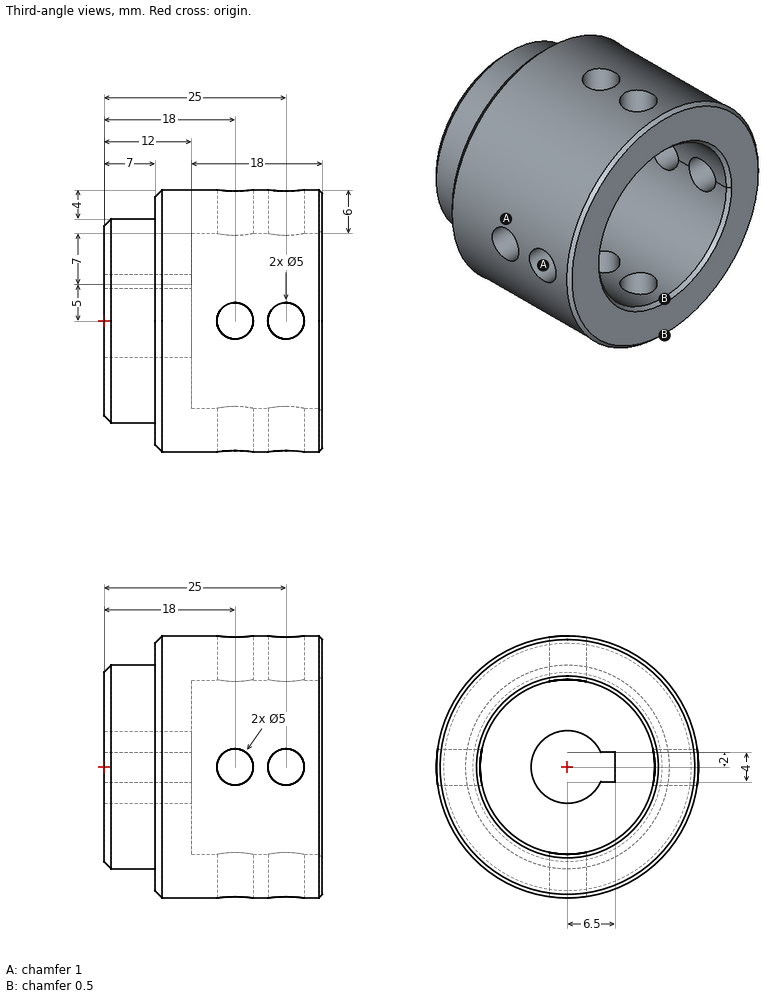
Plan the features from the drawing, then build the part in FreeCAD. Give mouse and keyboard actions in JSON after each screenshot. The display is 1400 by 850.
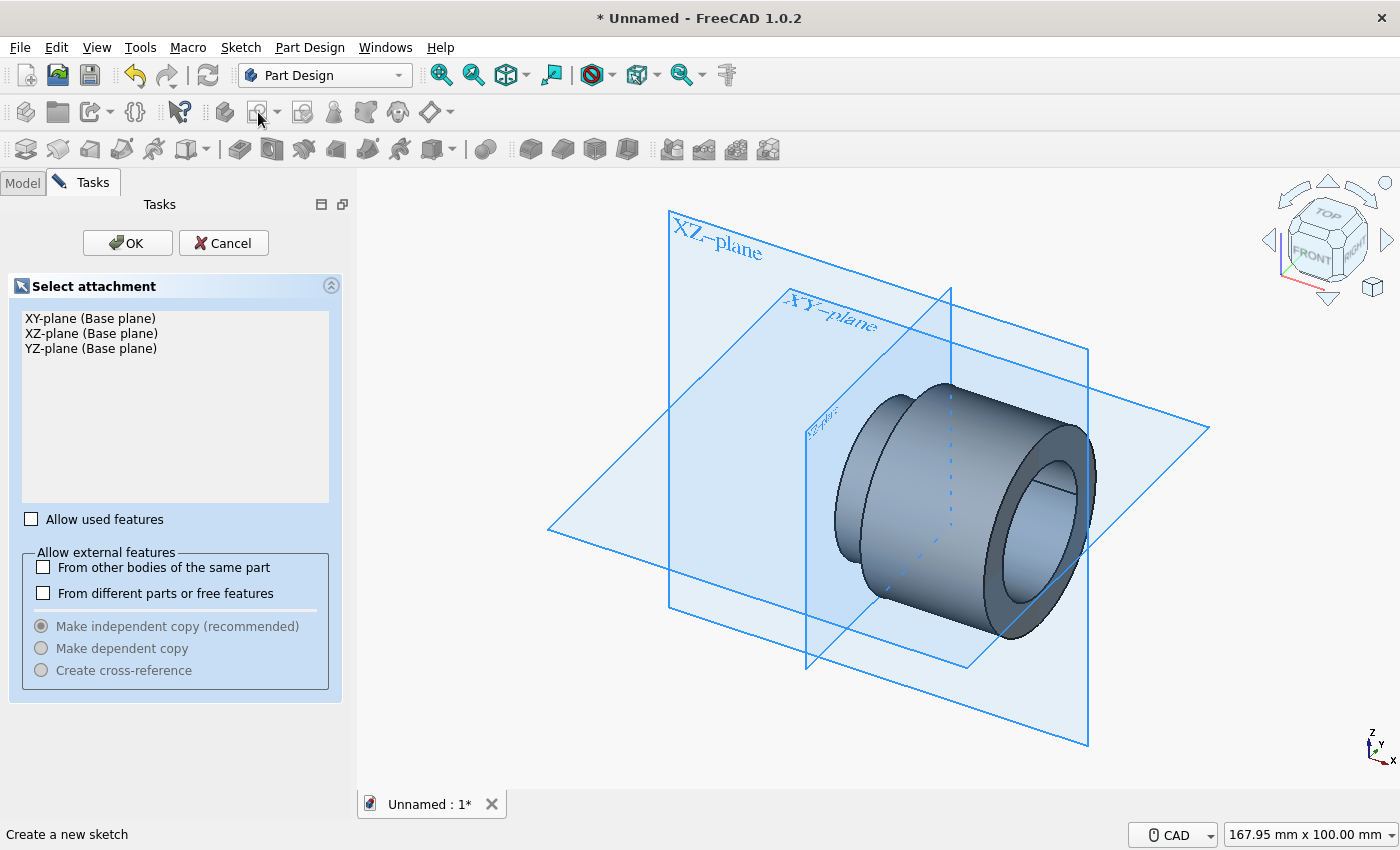
{"action": "left_click", "coordinate": [82, 348]}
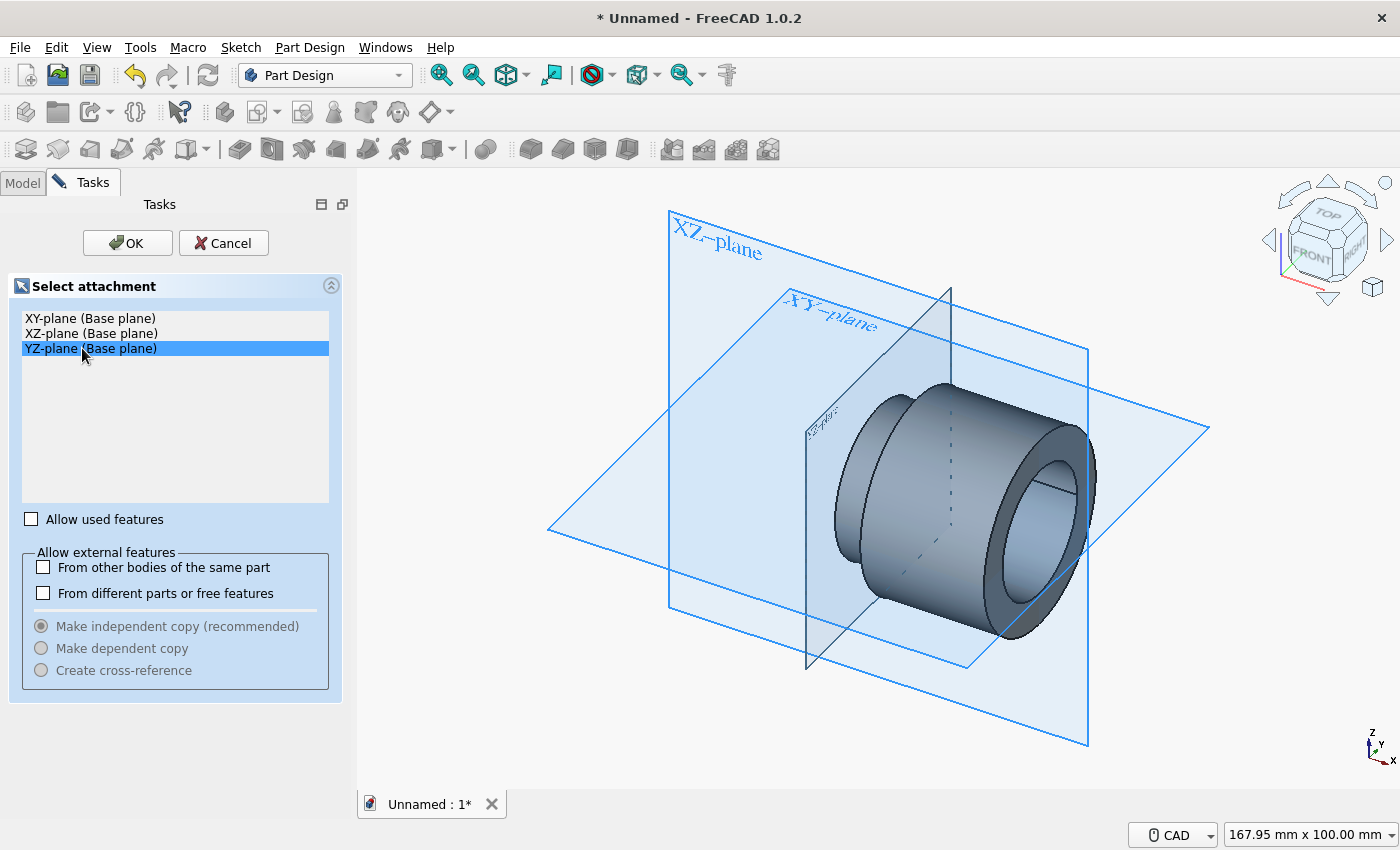
{"action": "left_click", "coordinate": [128, 243]}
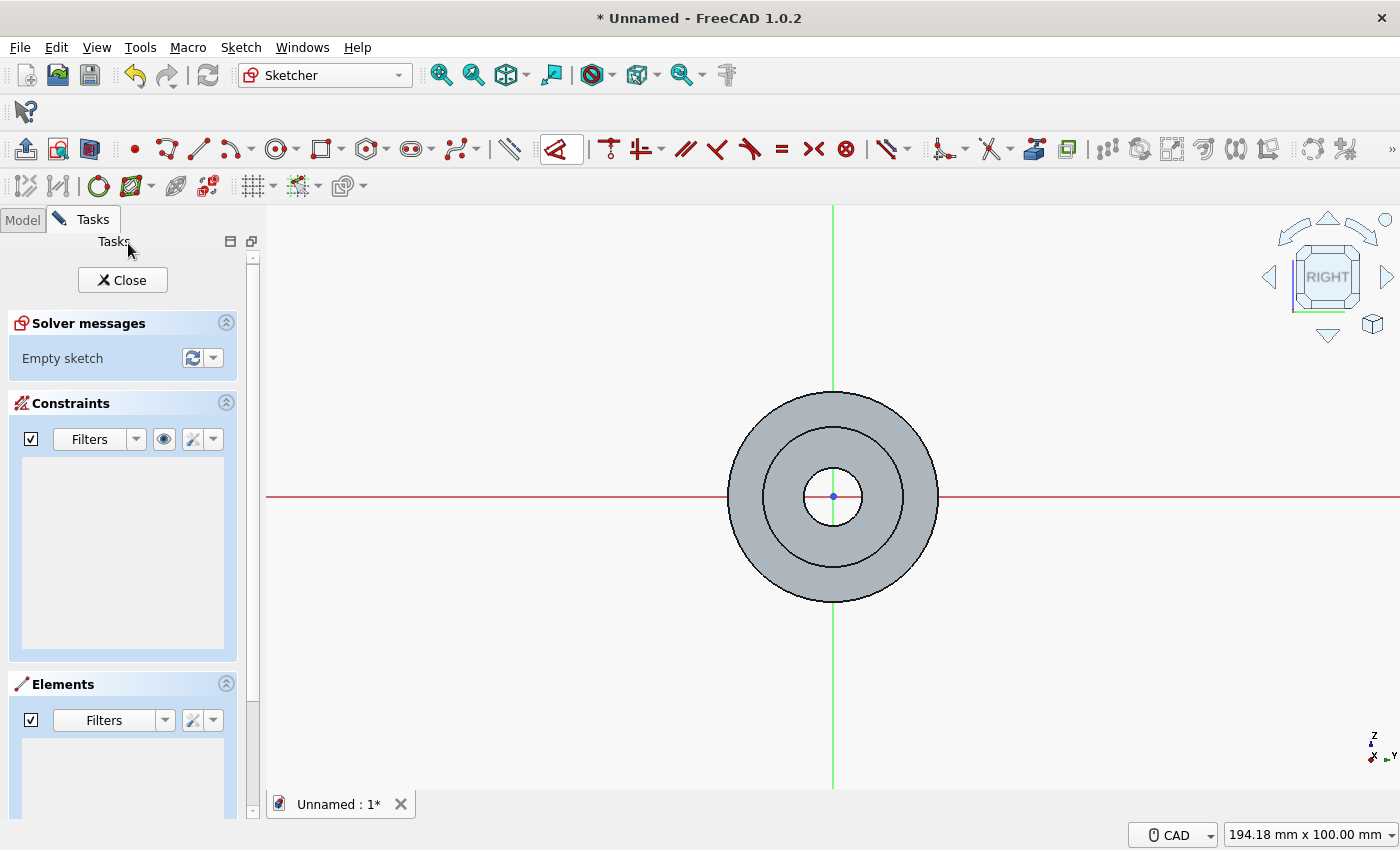
{"action": "left_click", "coordinate": [90, 150]}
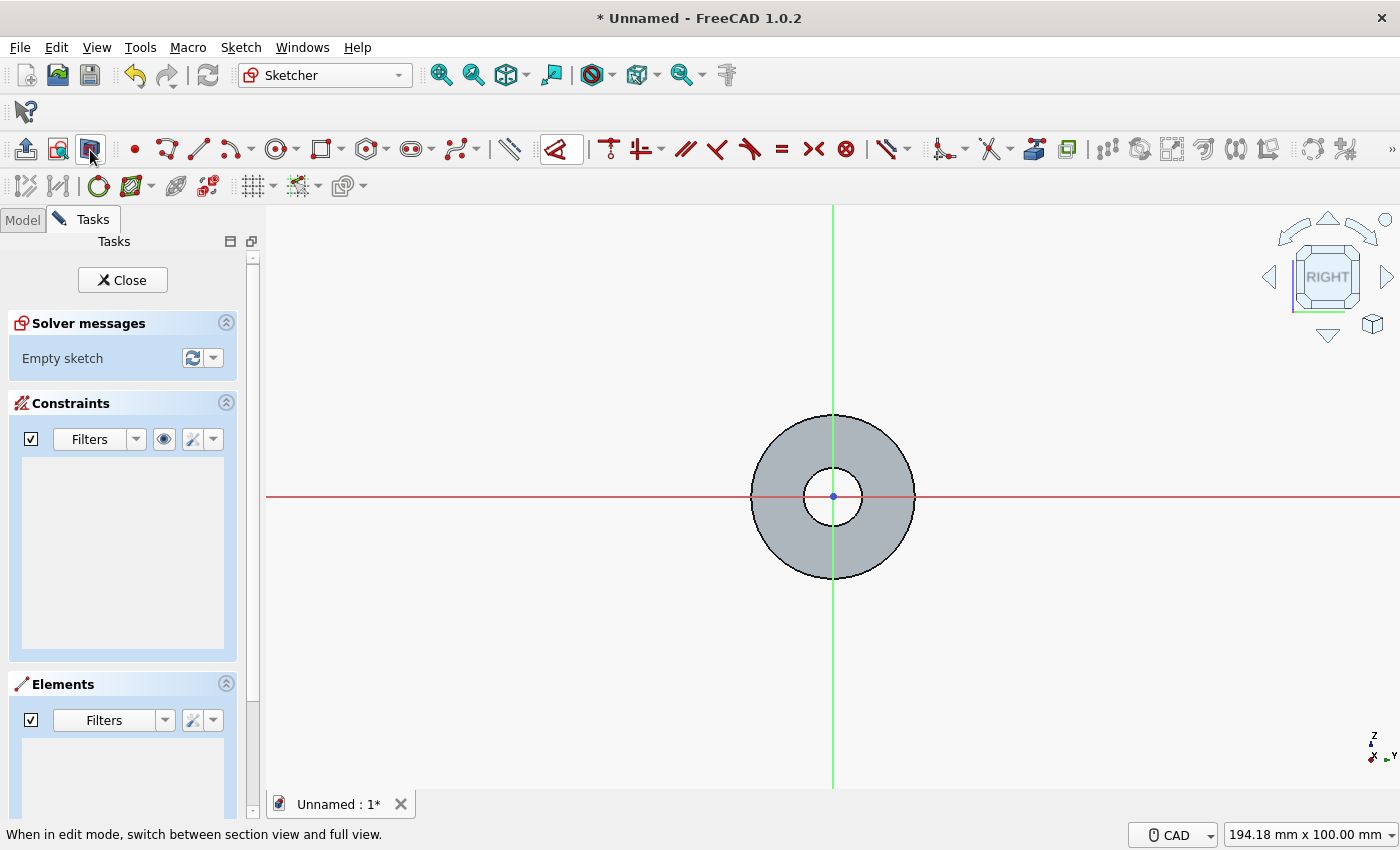
{"action": "scroll", "coordinate": [858, 497], "scroll_direction": "up", "scroll_amount": 14}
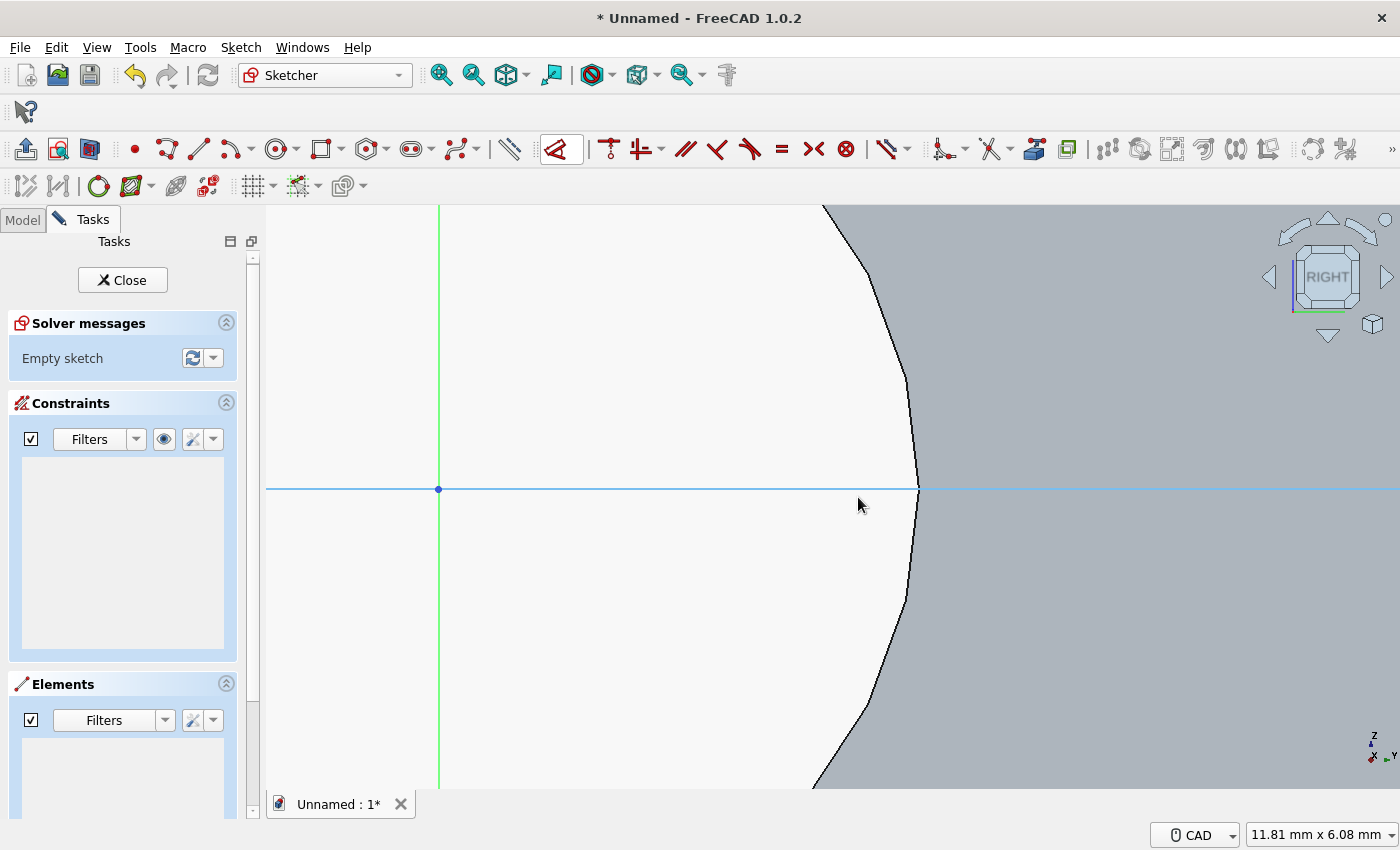
{"action": "left_click", "coordinate": [322, 150]}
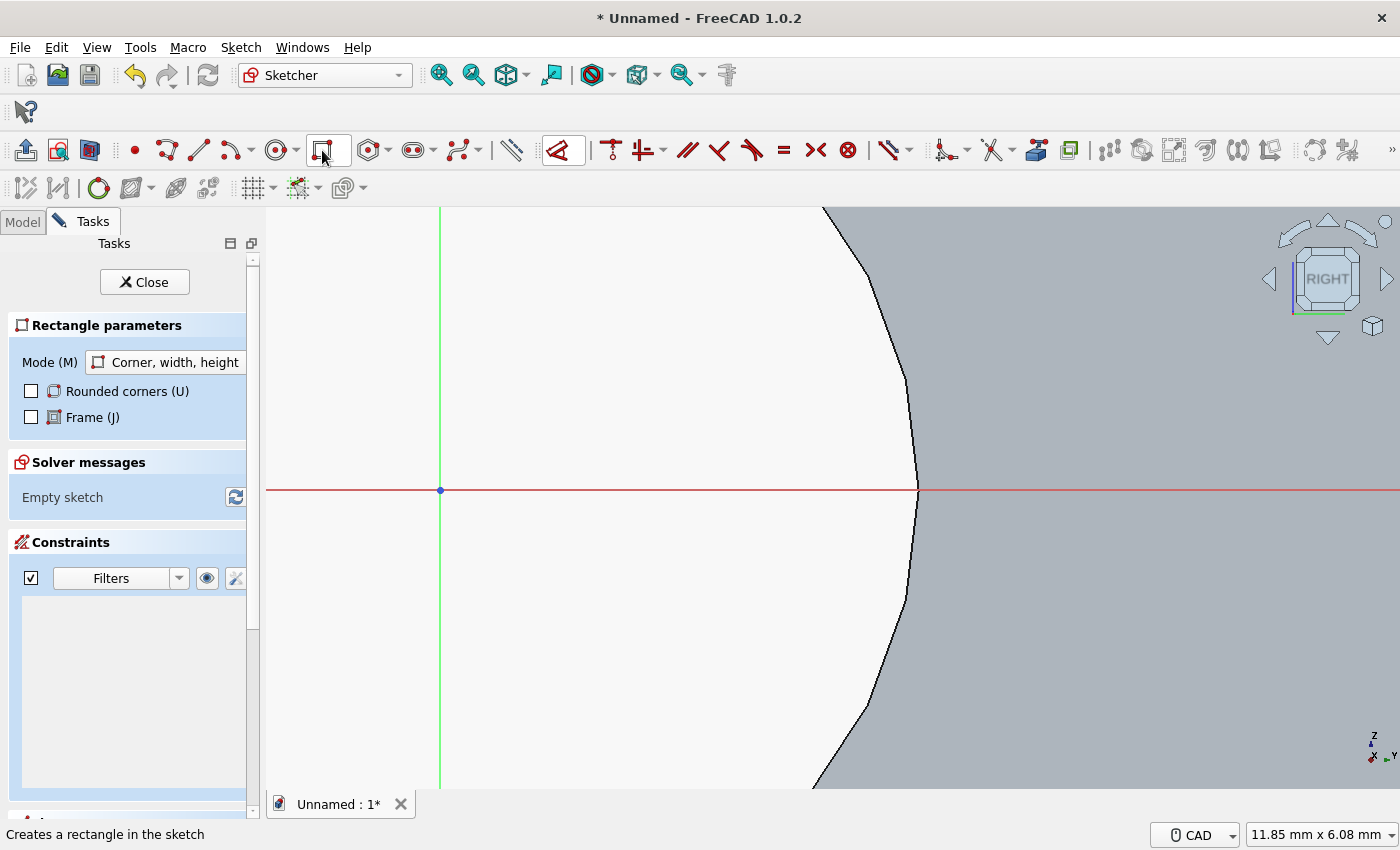
{"action": "left_click", "coordinate": [440, 299]}
{"action": "left_click", "coordinate": [1062, 682]}
{"action": "key", "text": "Escape"}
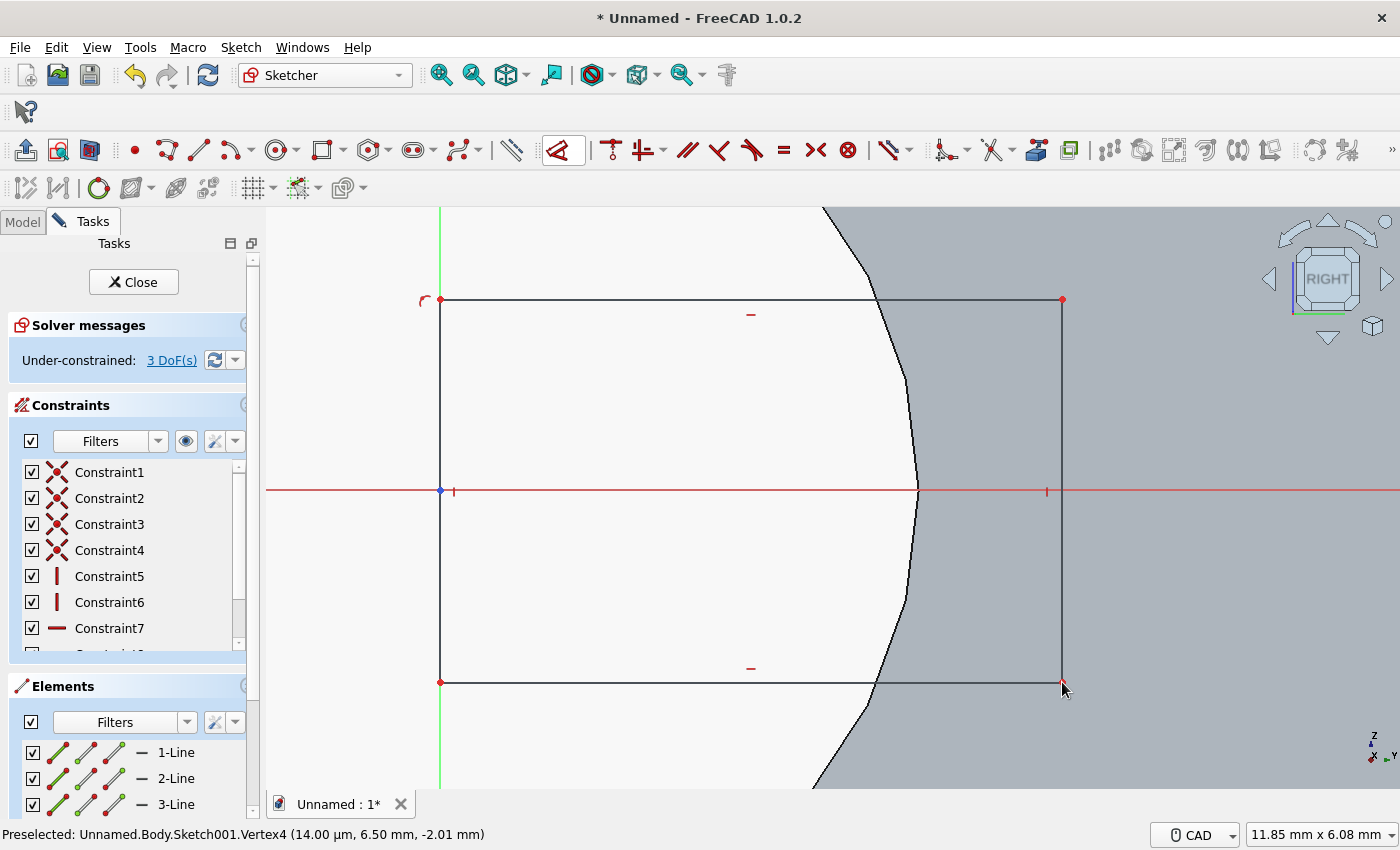
{"action": "left_click", "coordinate": [440, 415]}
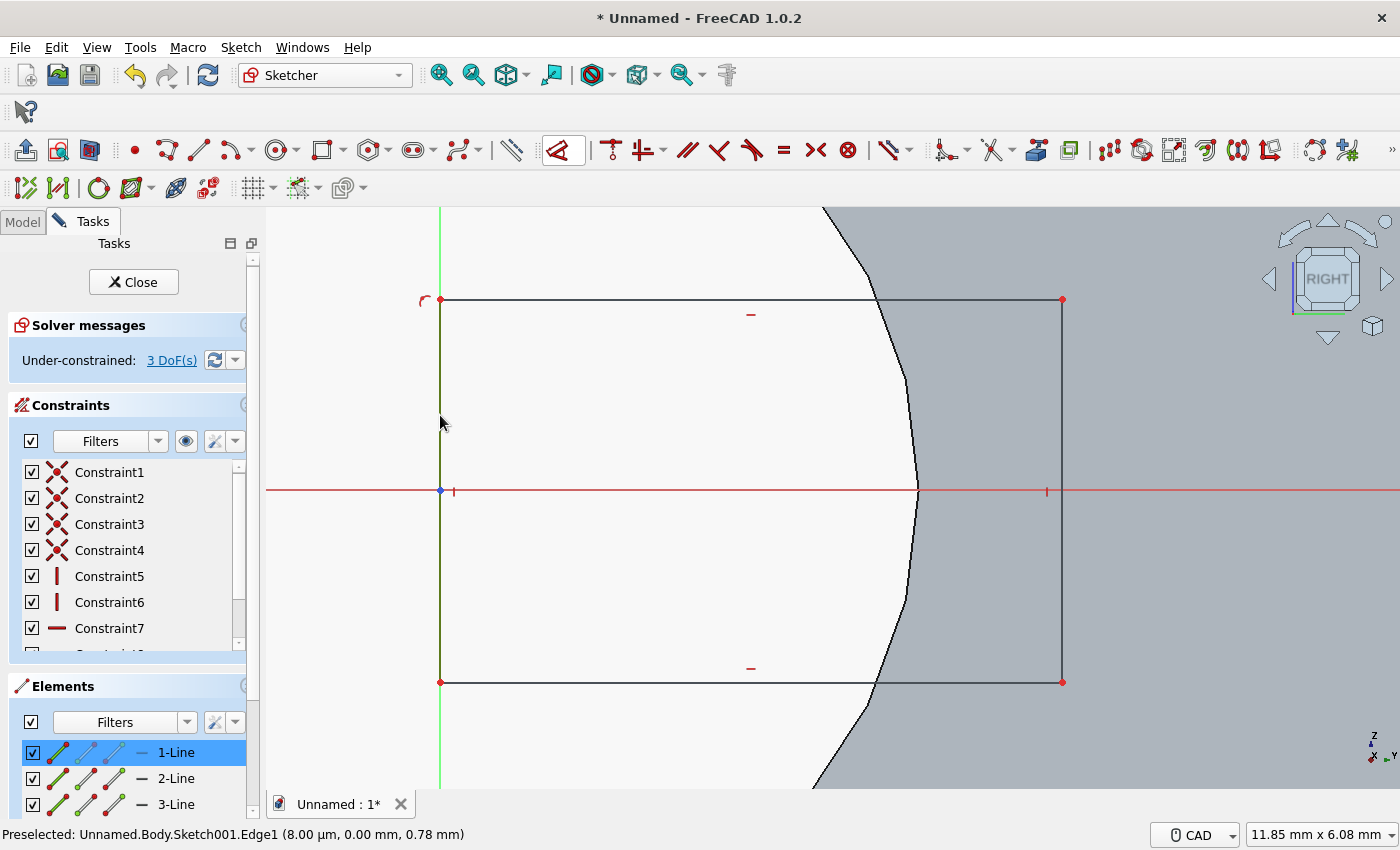
{"action": "left_click", "coordinate": [580, 150]}